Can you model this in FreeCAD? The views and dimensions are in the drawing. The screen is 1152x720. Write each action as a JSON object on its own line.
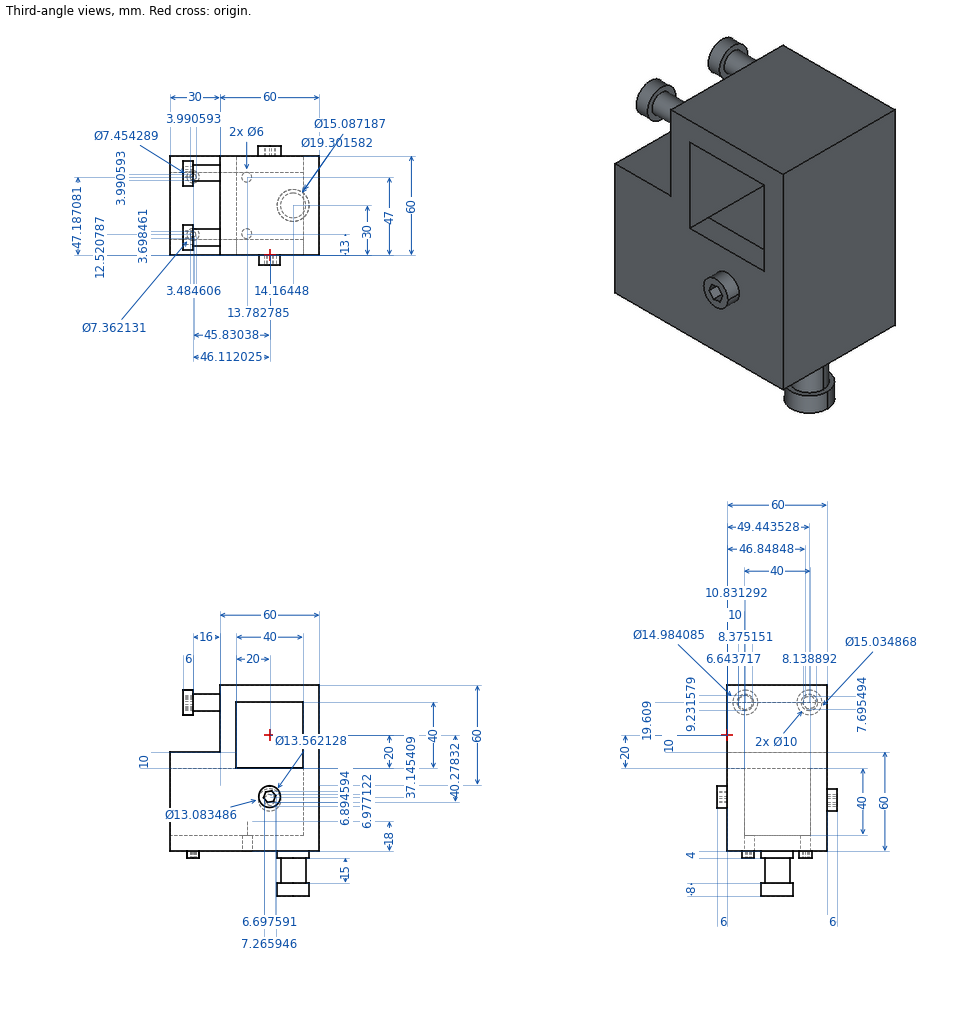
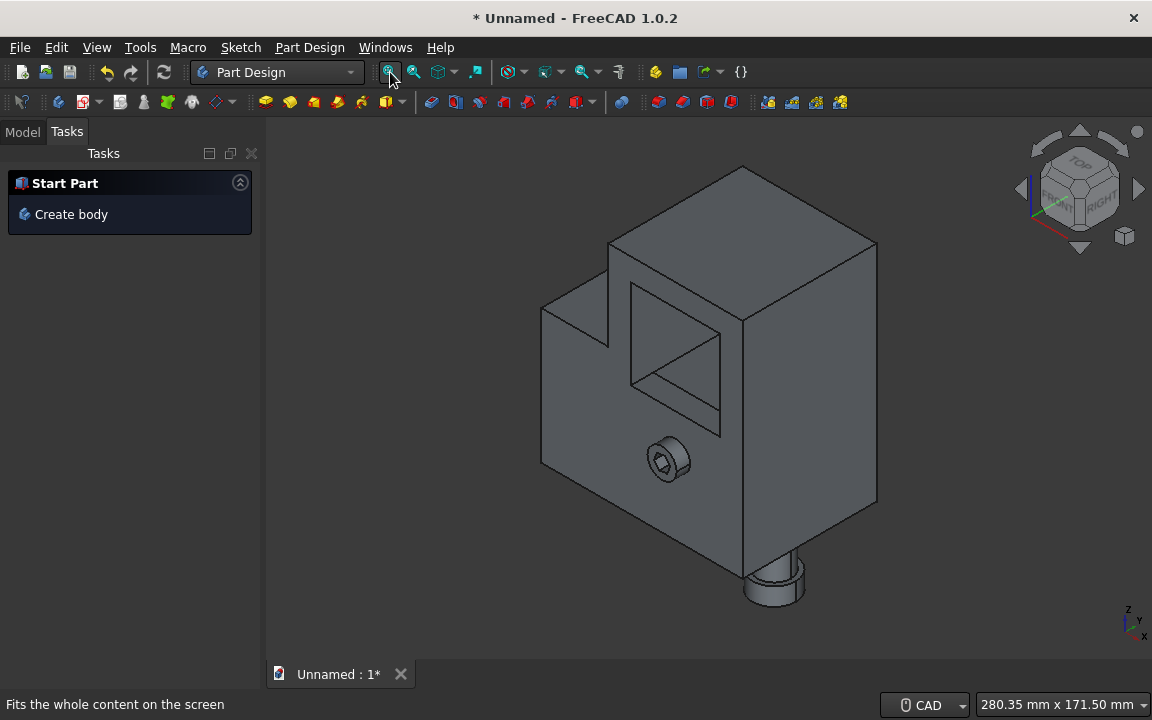
{"action": "key", "text": "6"}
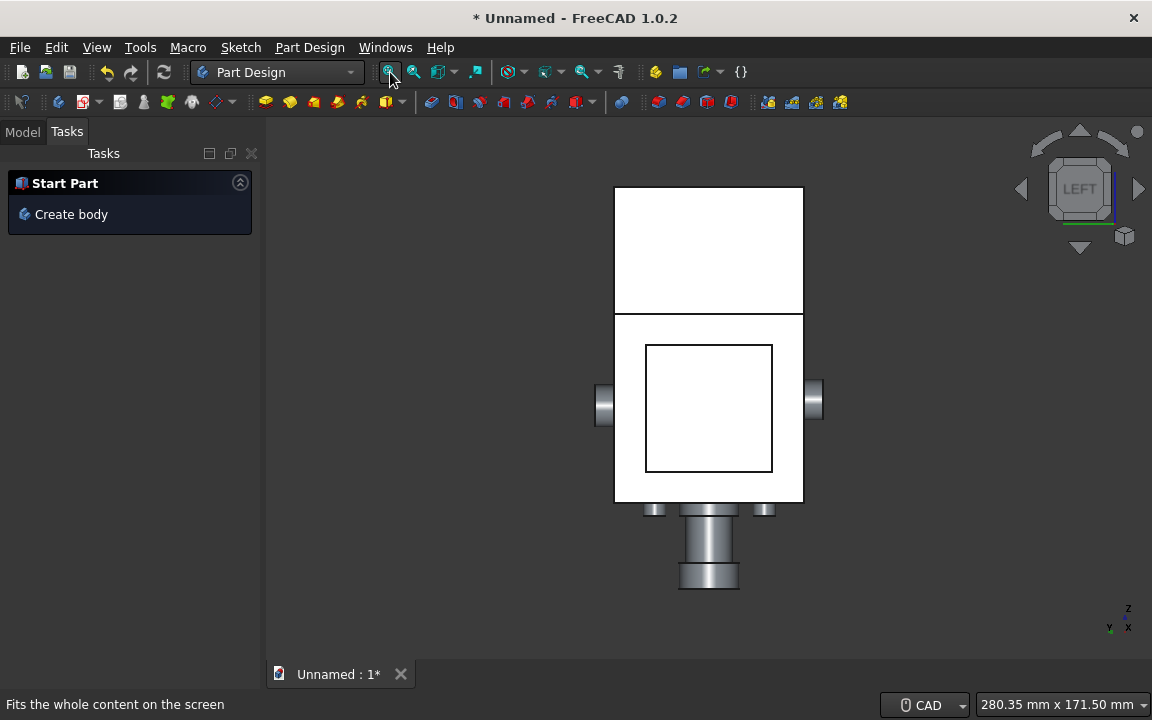
{"action": "left_click", "coordinate": [682, 250]}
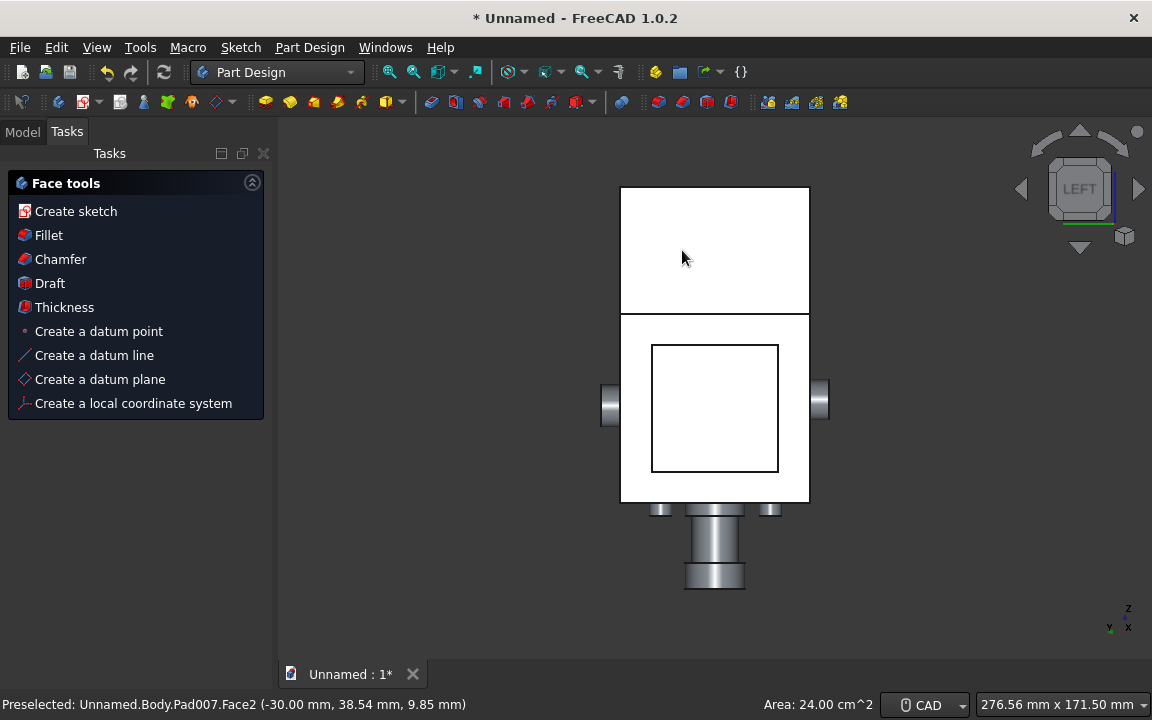
{"action": "left_click", "coordinate": [84, 102]}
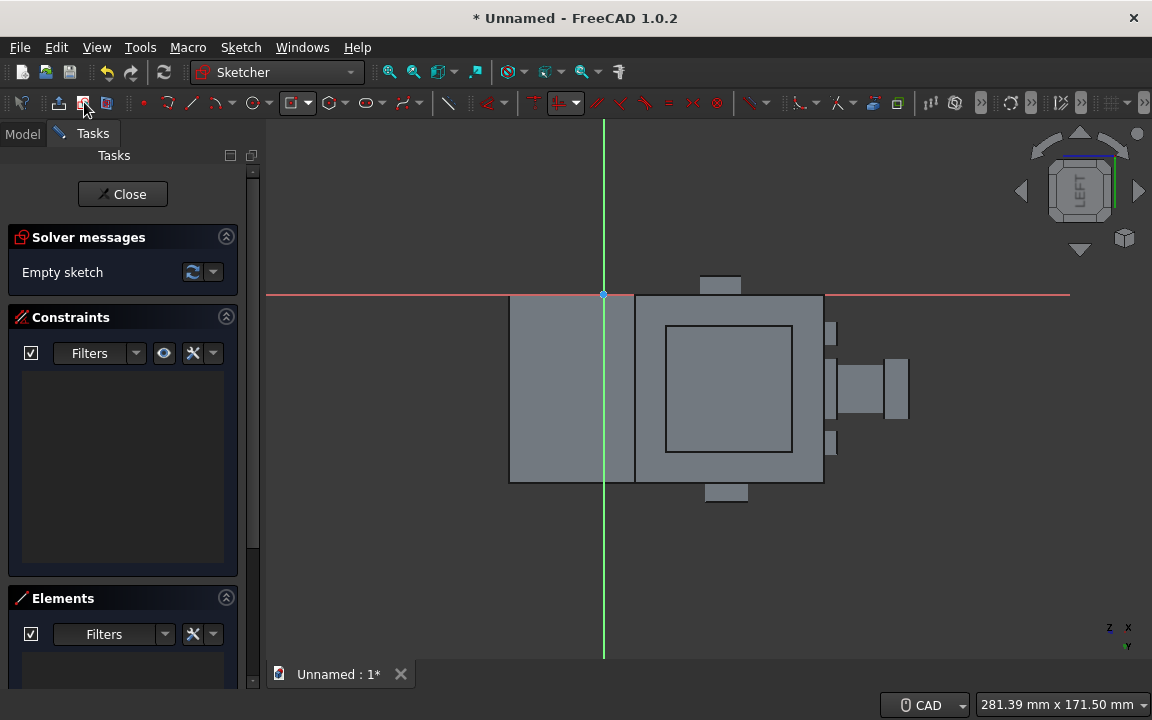
{"action": "scroll", "coordinate": [473, 370], "scroll_direction": "up", "scroll_amount": 3}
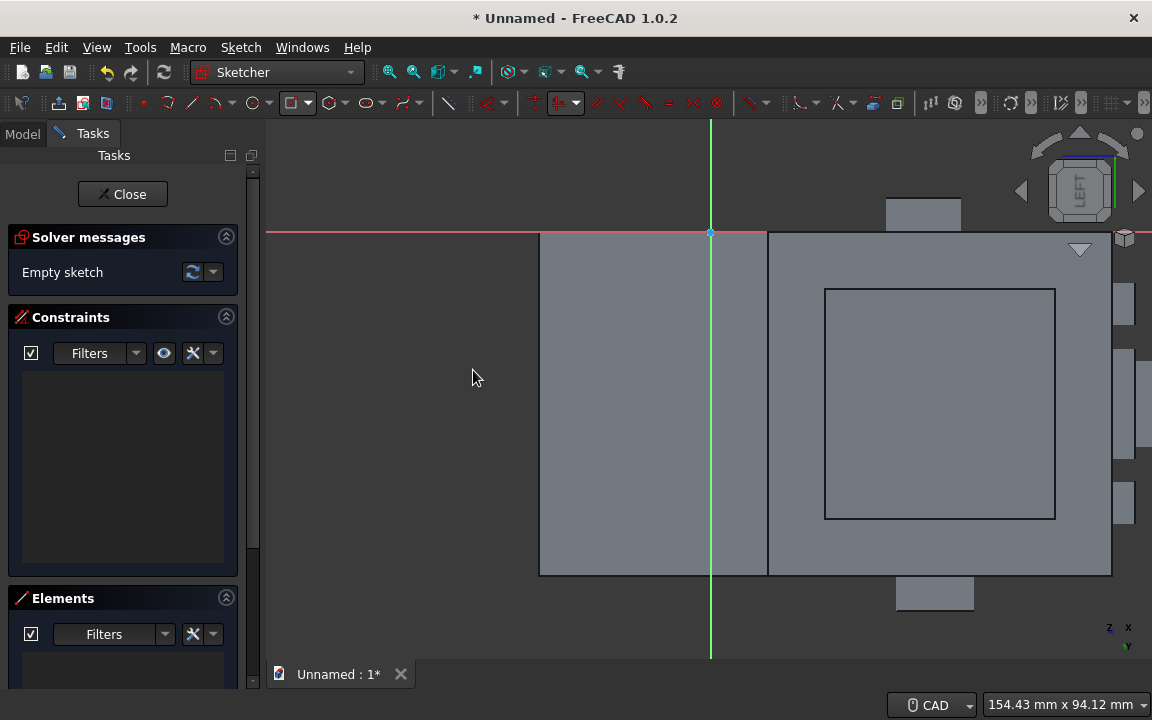
{"action": "left_click", "coordinate": [254, 104]}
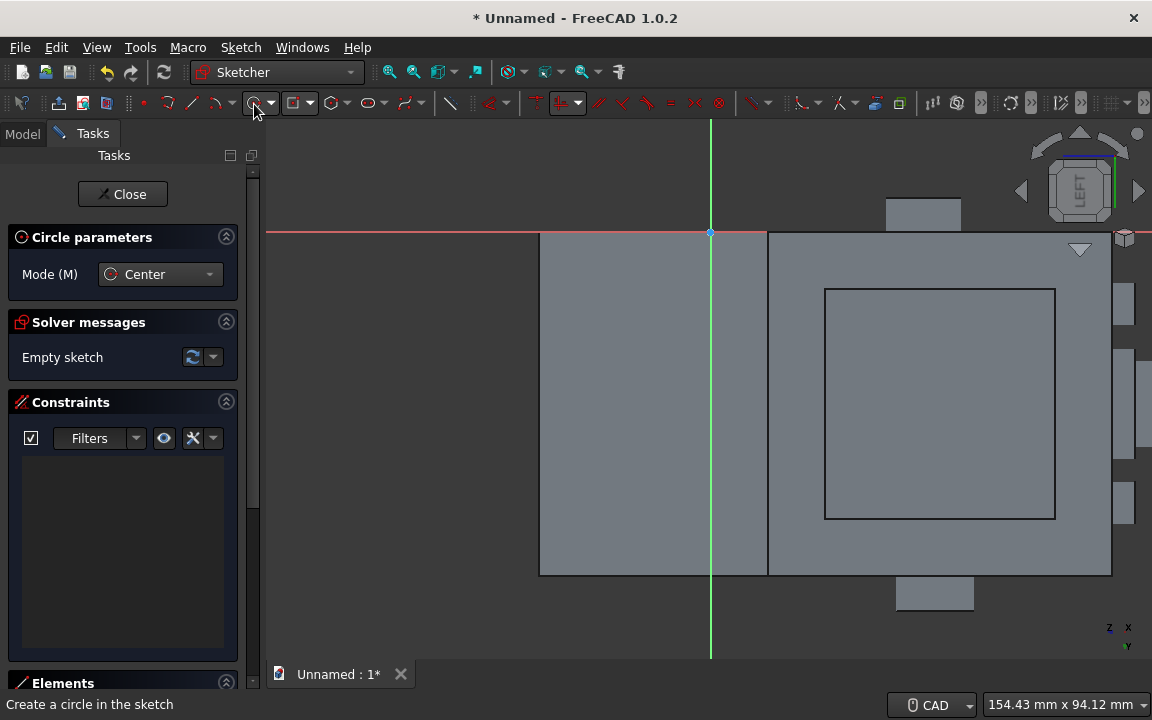
{"action": "left_click", "coordinate": [598, 516]}
{"action": "left_click", "coordinate": [618, 496]}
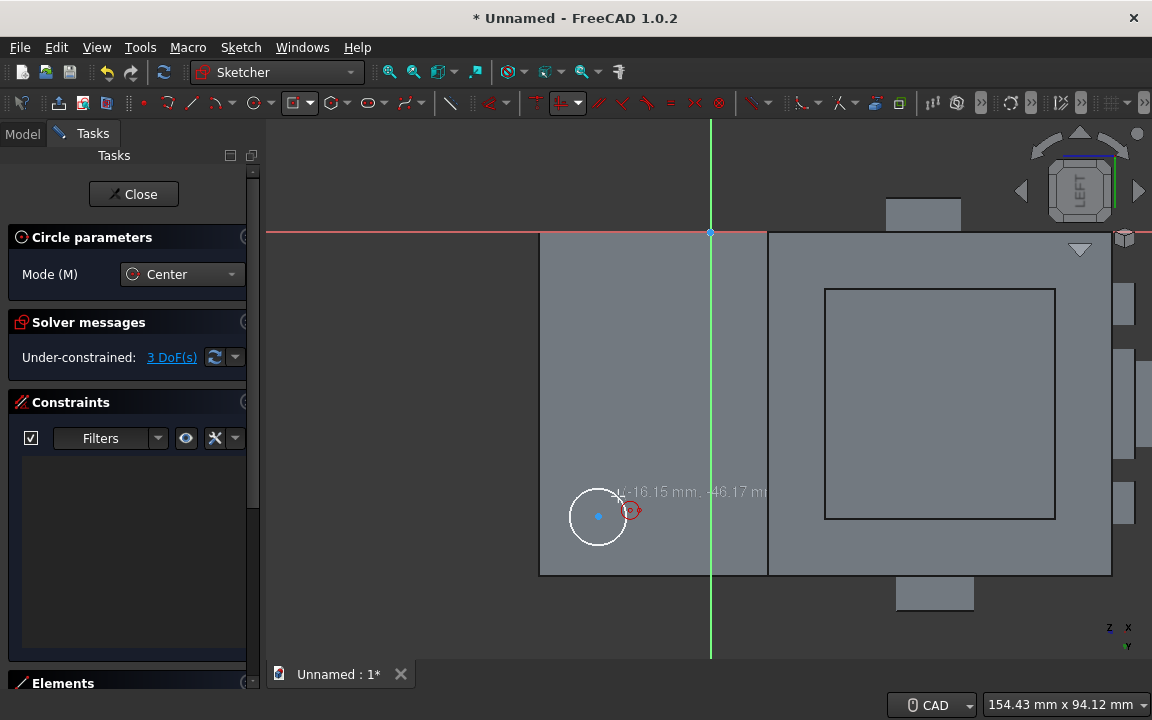
{"action": "left_click", "coordinate": [598, 294]}
{"action": "left_click", "coordinate": [618, 274]}
{"action": "key", "text": "Escape"}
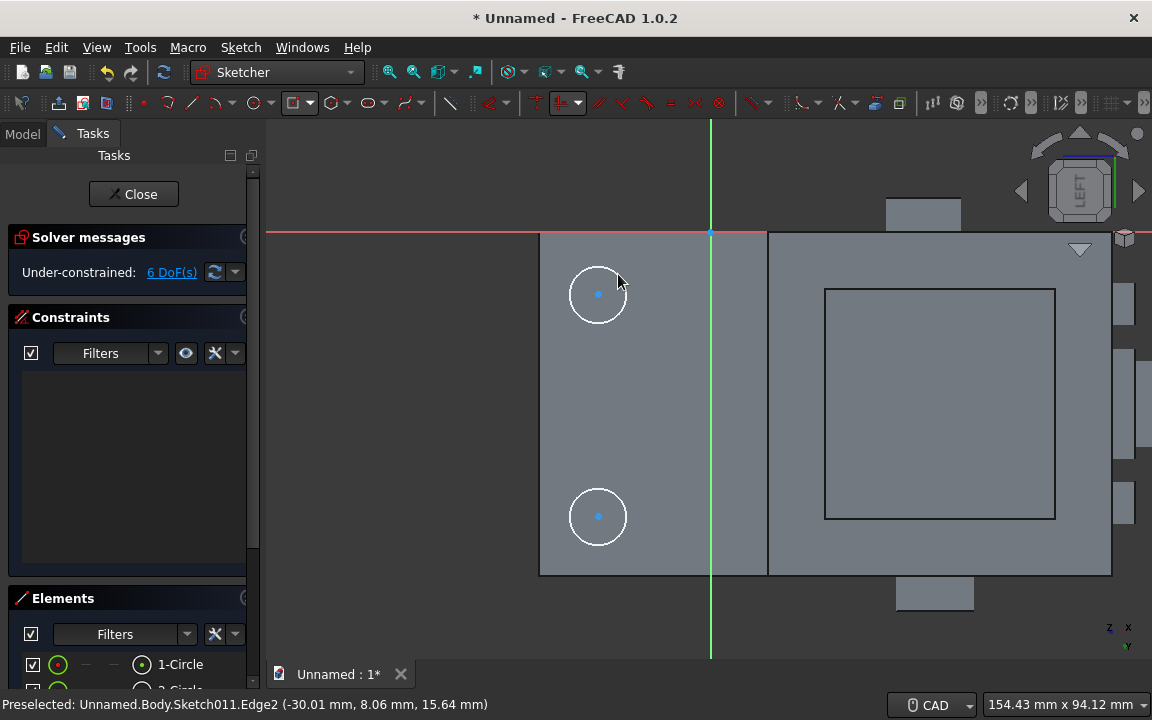
{"action": "left_click", "coordinate": [618, 497]}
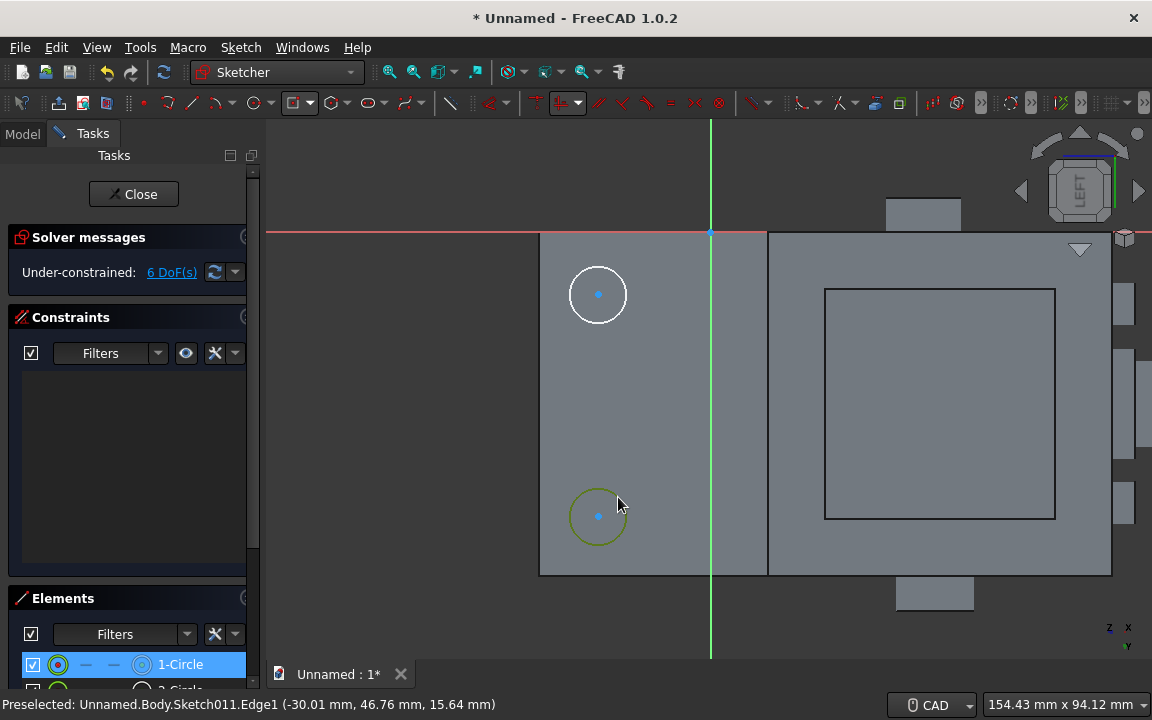
{"action": "left_click", "coordinate": [618, 275]}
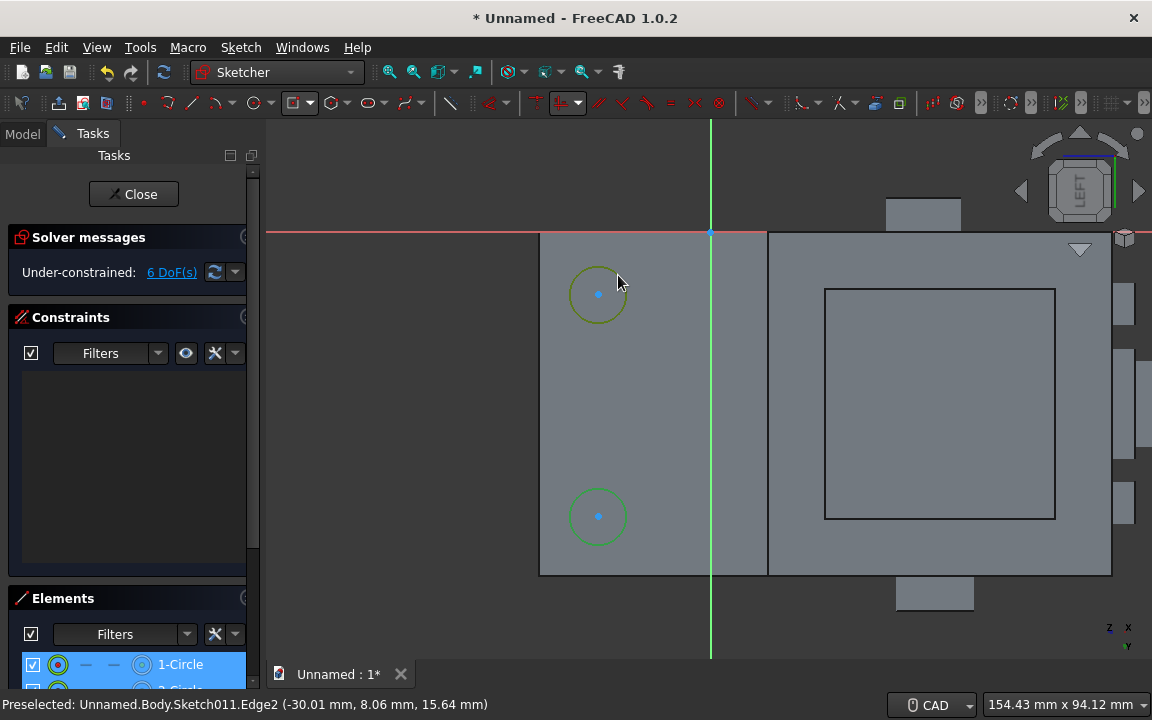
{"action": "left_click", "coordinate": [672, 104]}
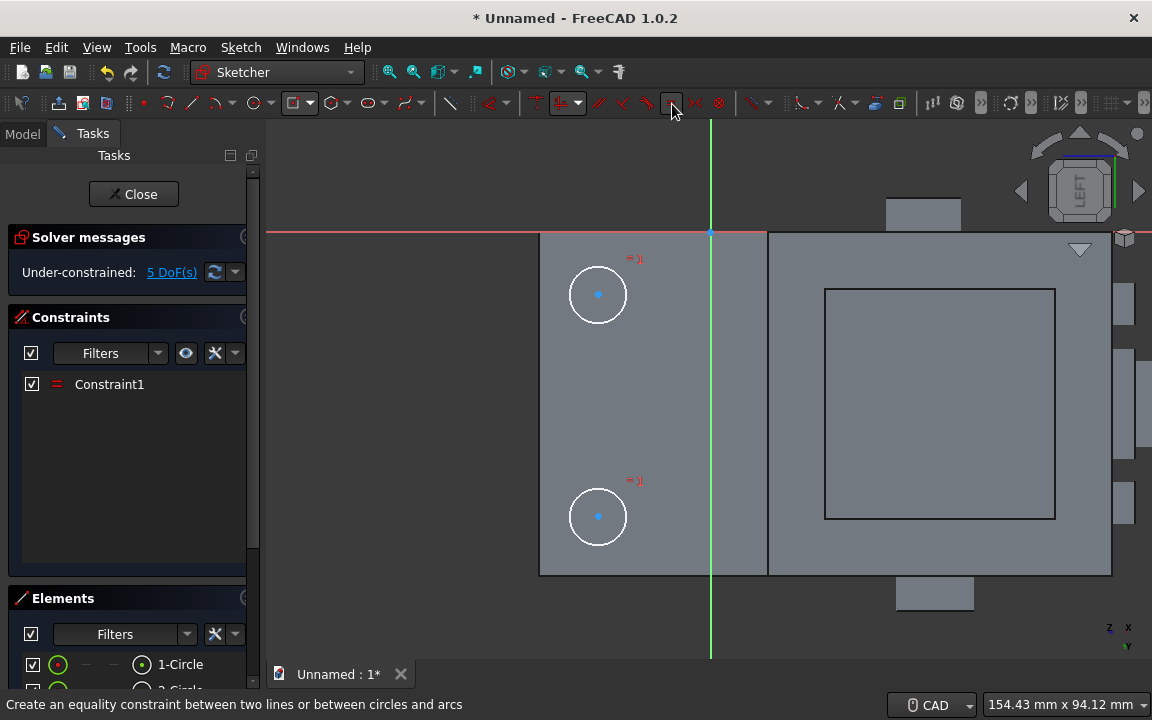
{"action": "left_click", "coordinate": [598, 517]}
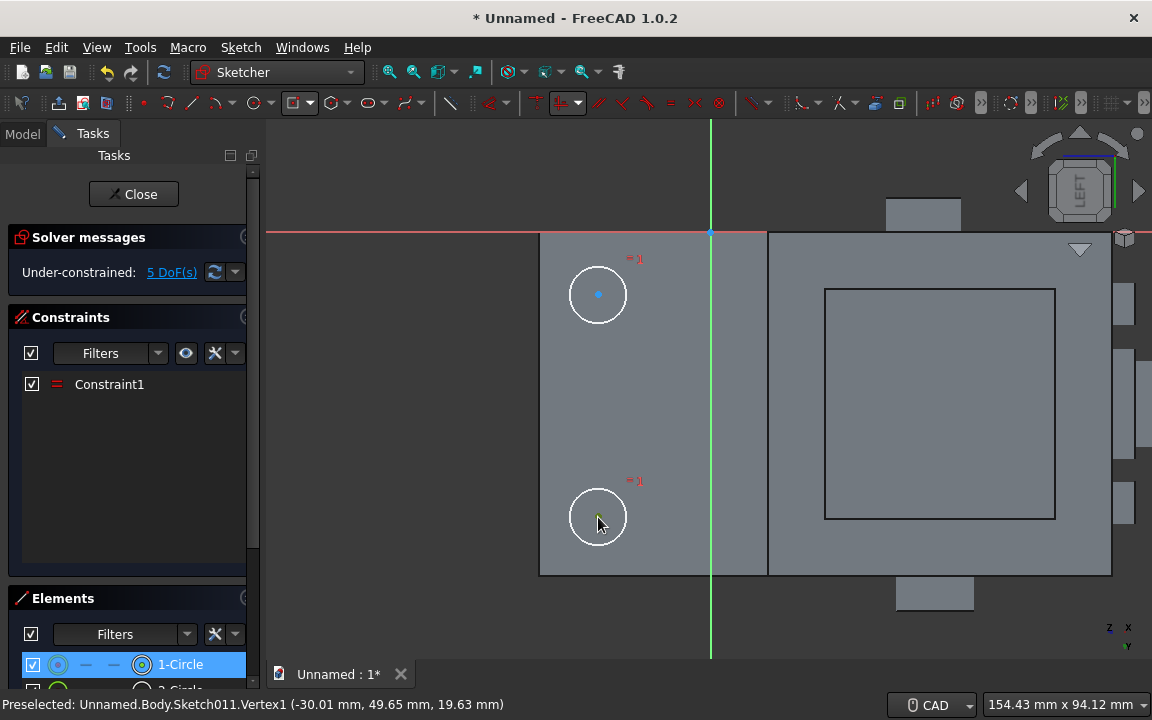
{"action": "left_click", "coordinate": [598, 295]}